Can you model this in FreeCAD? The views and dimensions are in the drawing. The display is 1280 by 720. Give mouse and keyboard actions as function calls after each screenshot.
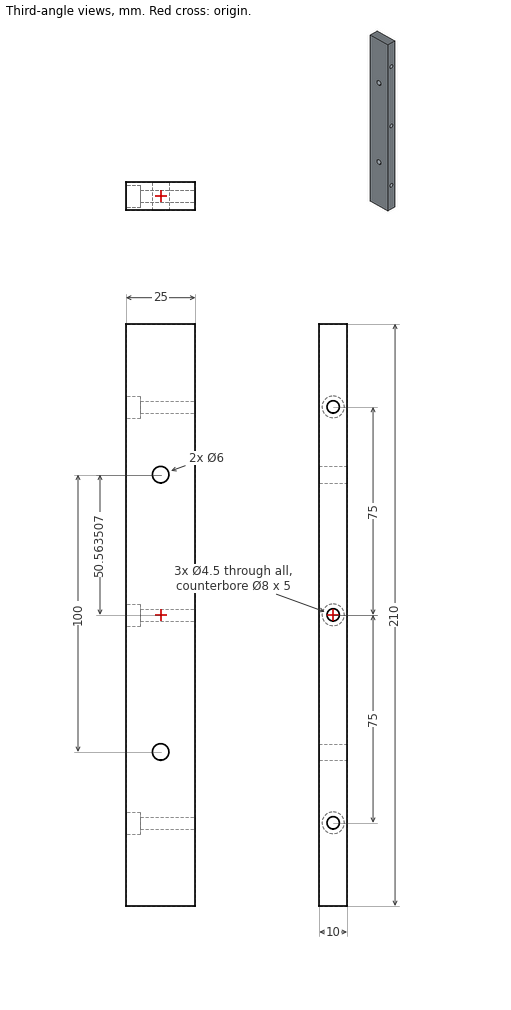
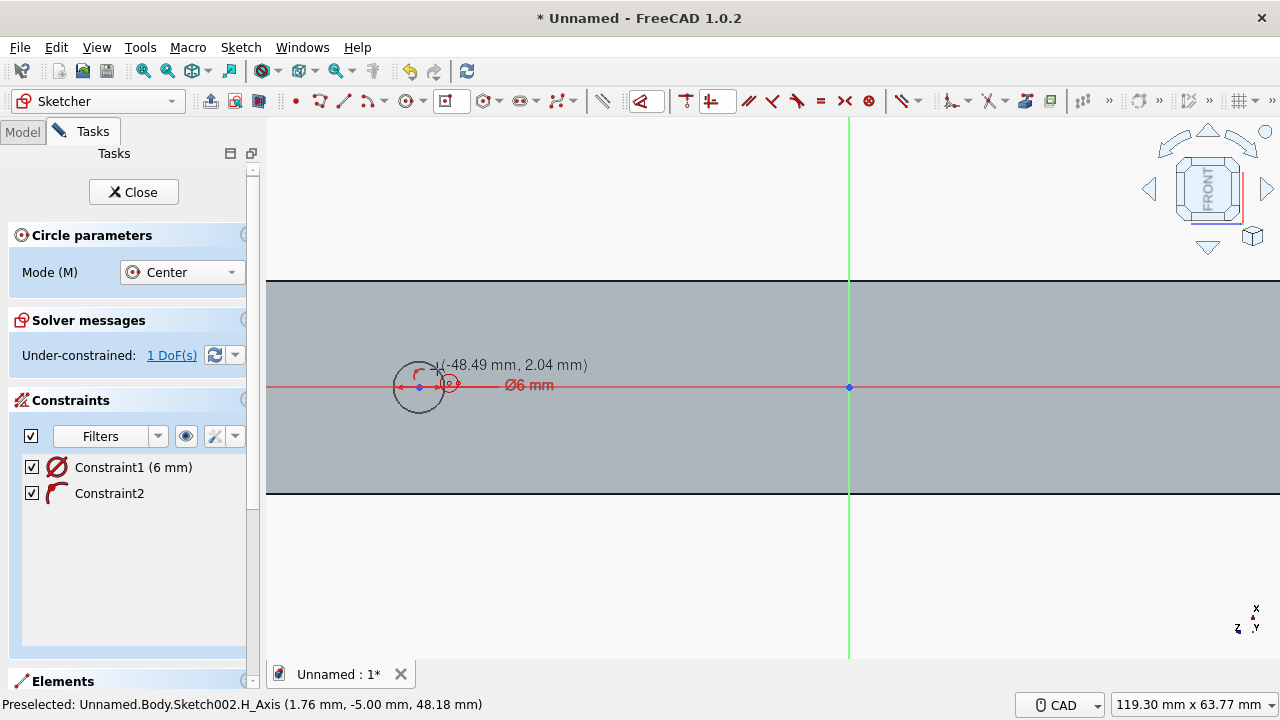
scroll(420, 389, down, 2)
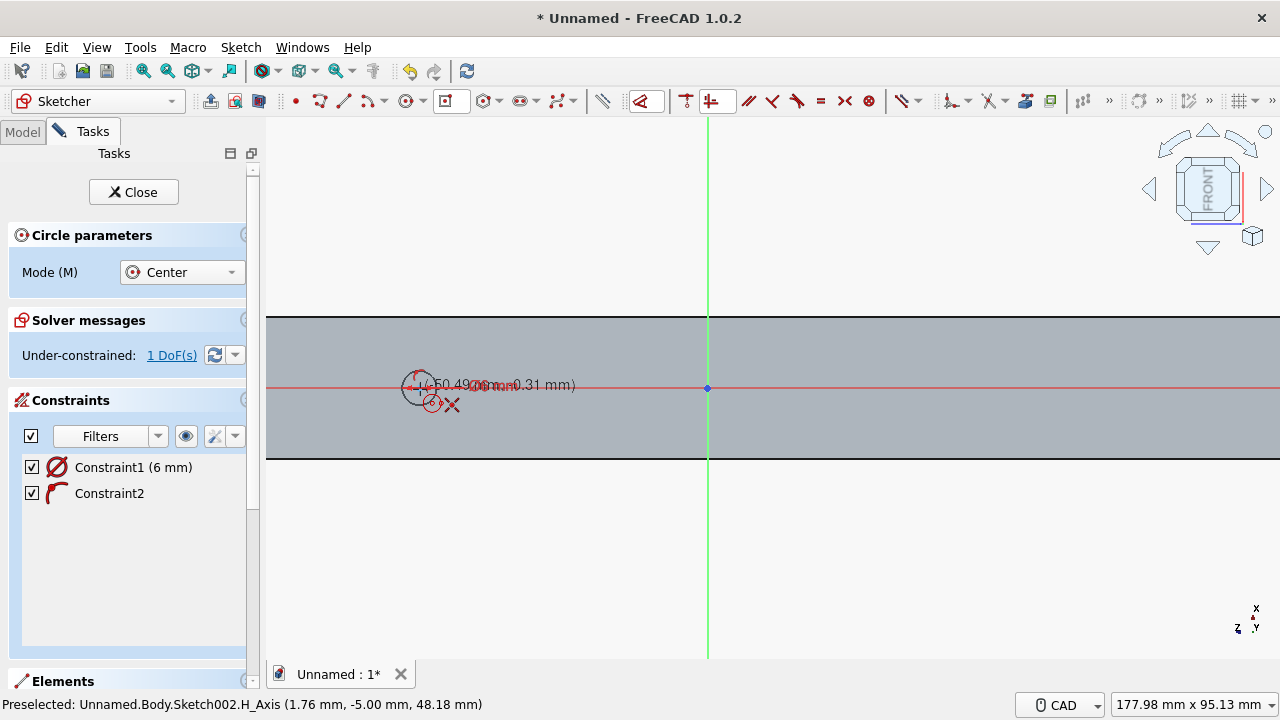
scroll(989, 388, up, 2)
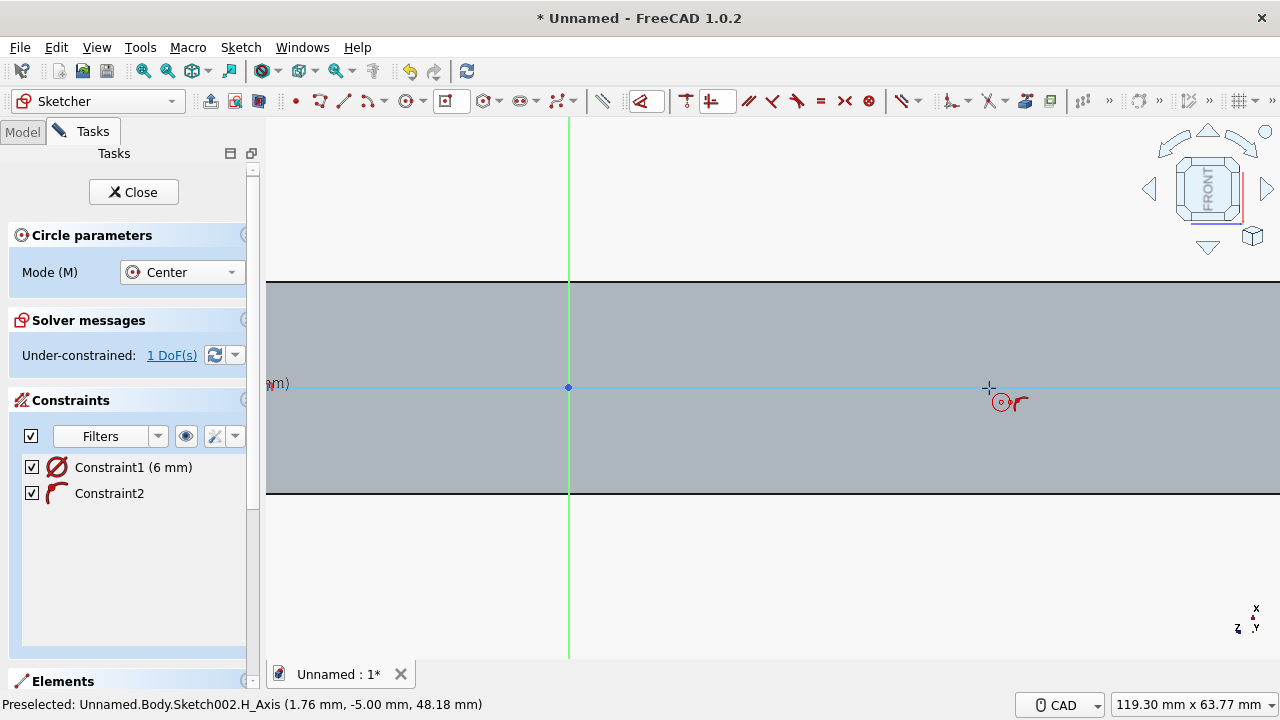
click(989, 388)
move(1007, 370)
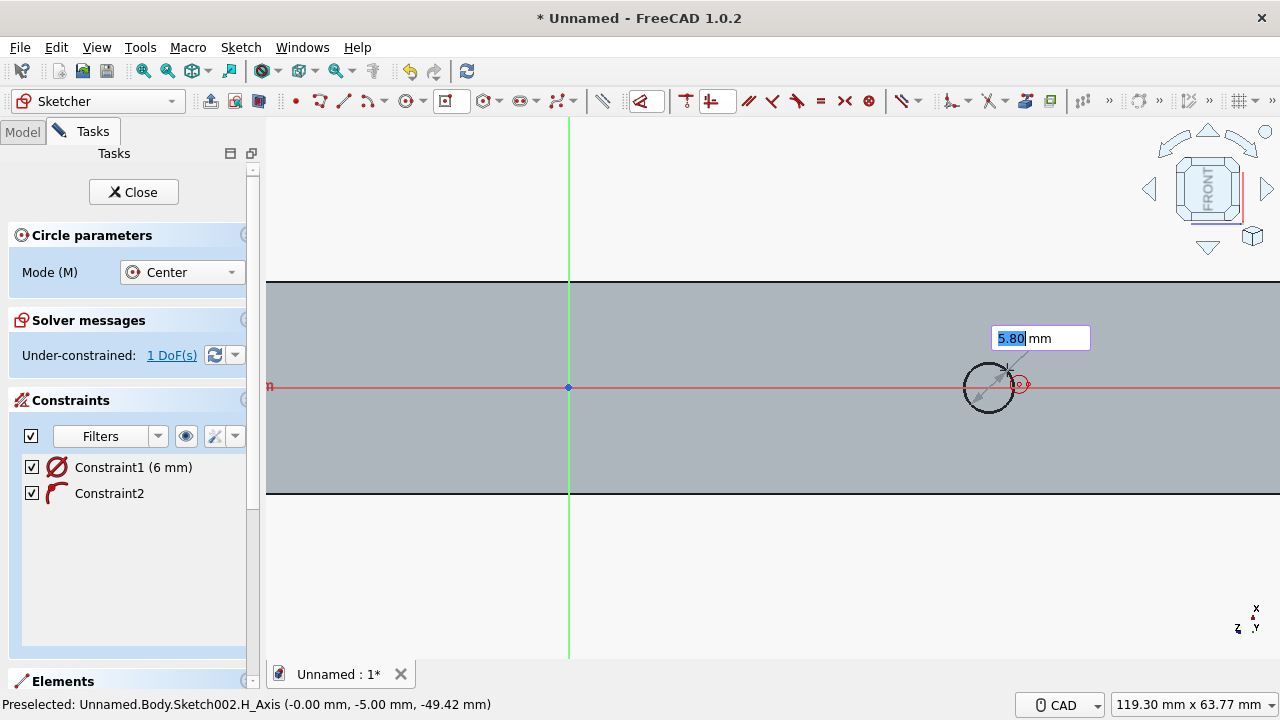
text(6)
key(Return)
key(Escape)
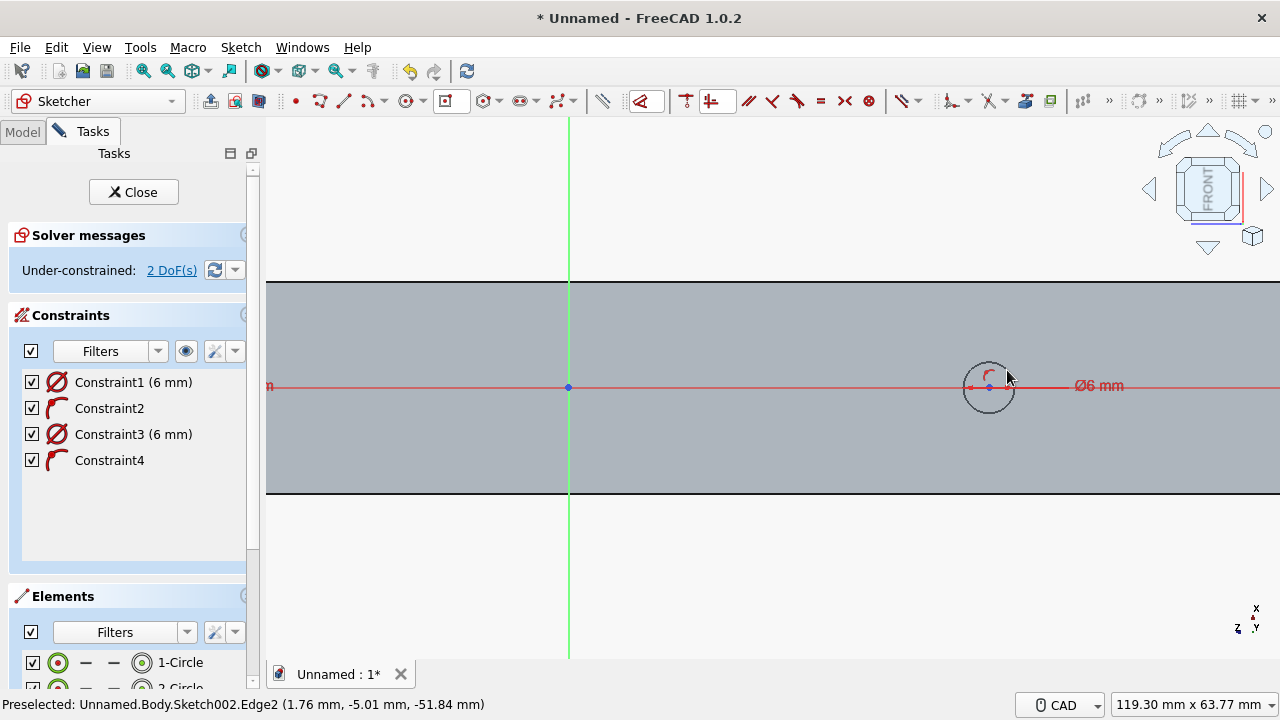
scroll(990, 388, down, 2)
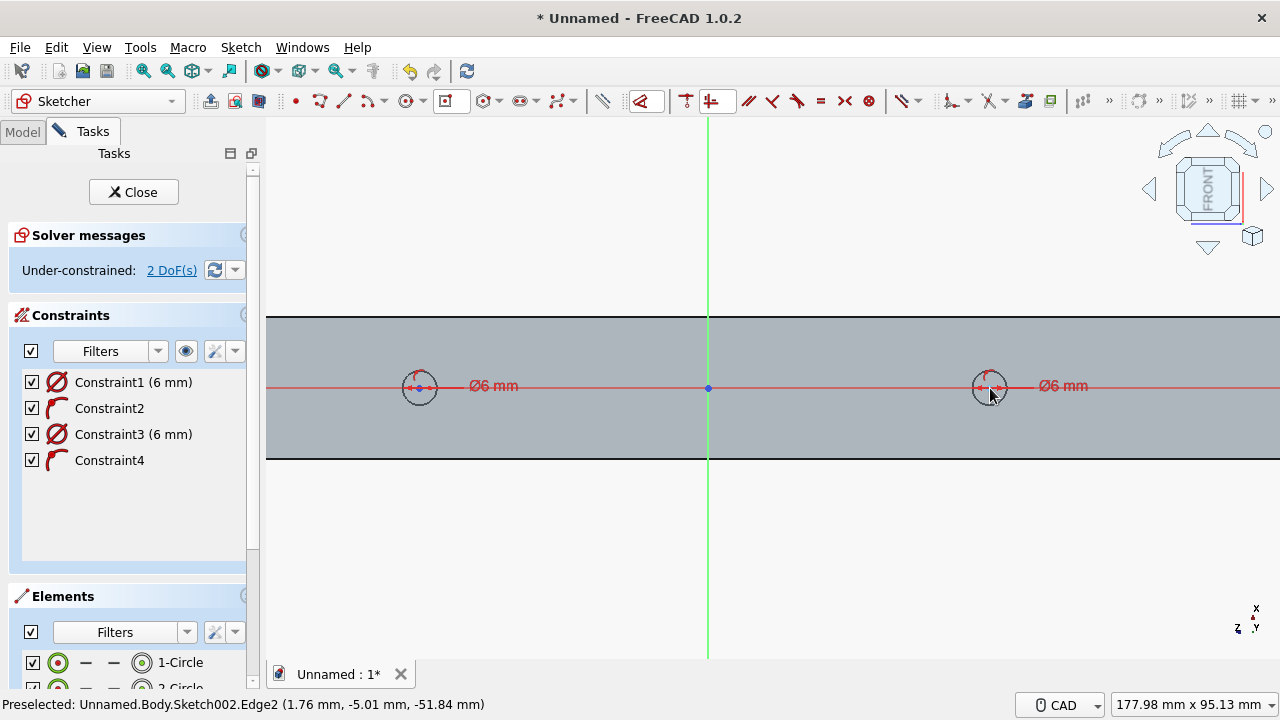
click(420, 388)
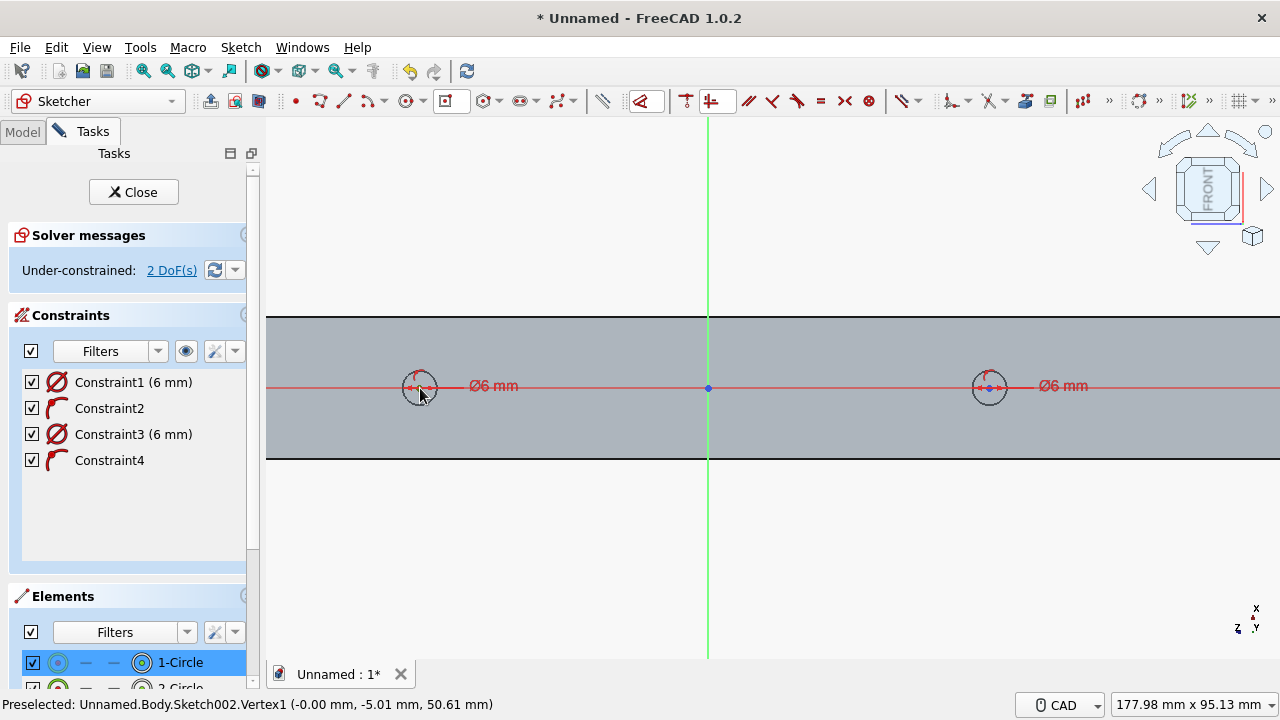
click(990, 388)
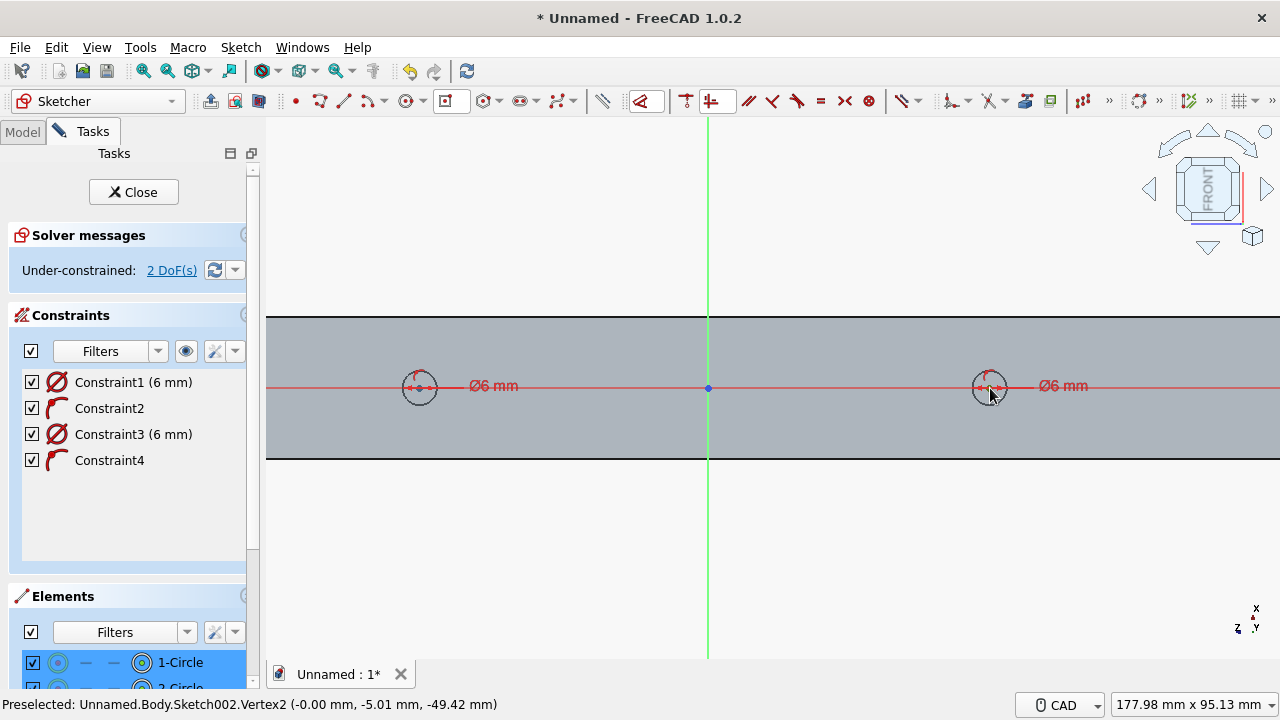
key(l)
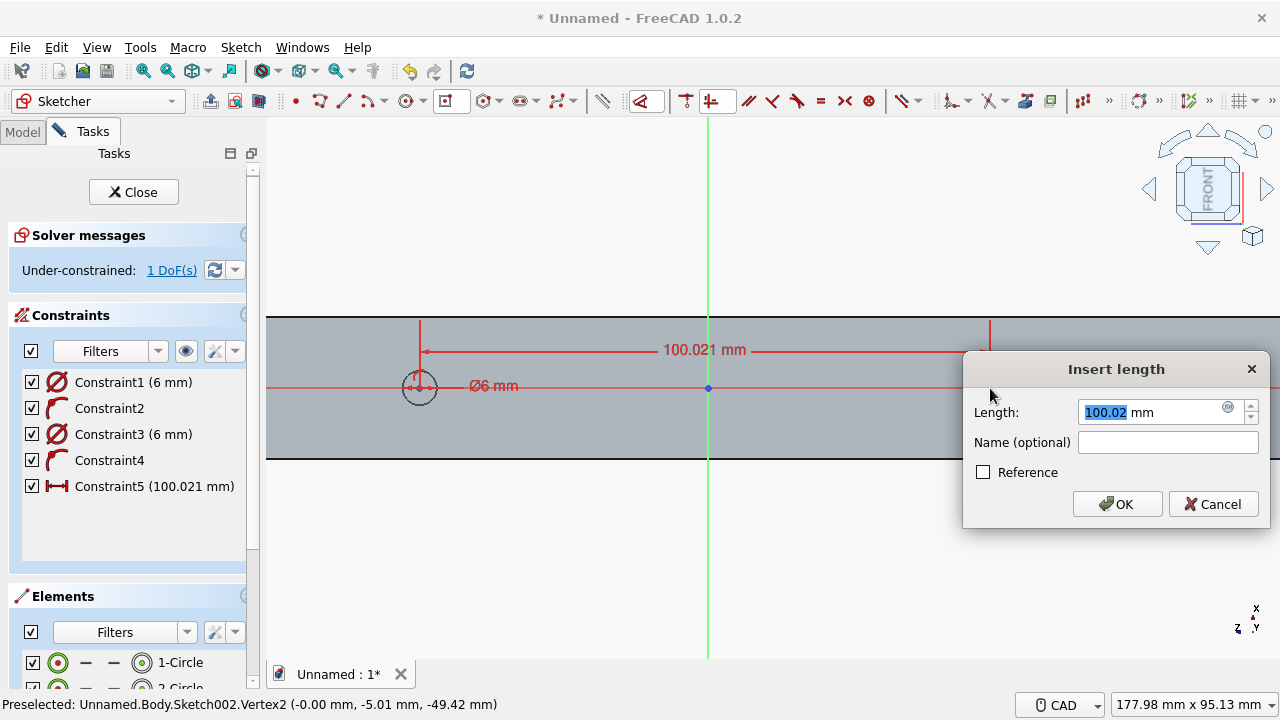
text(100)
key(Return)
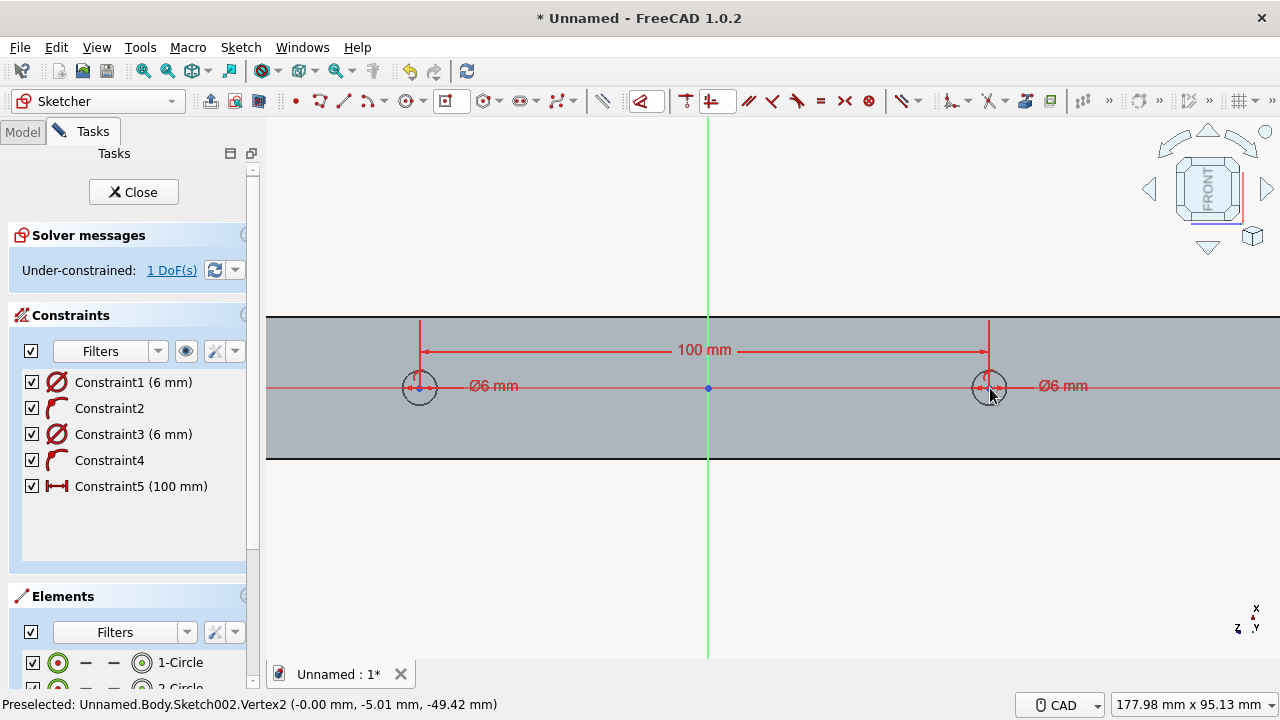
click(420, 388)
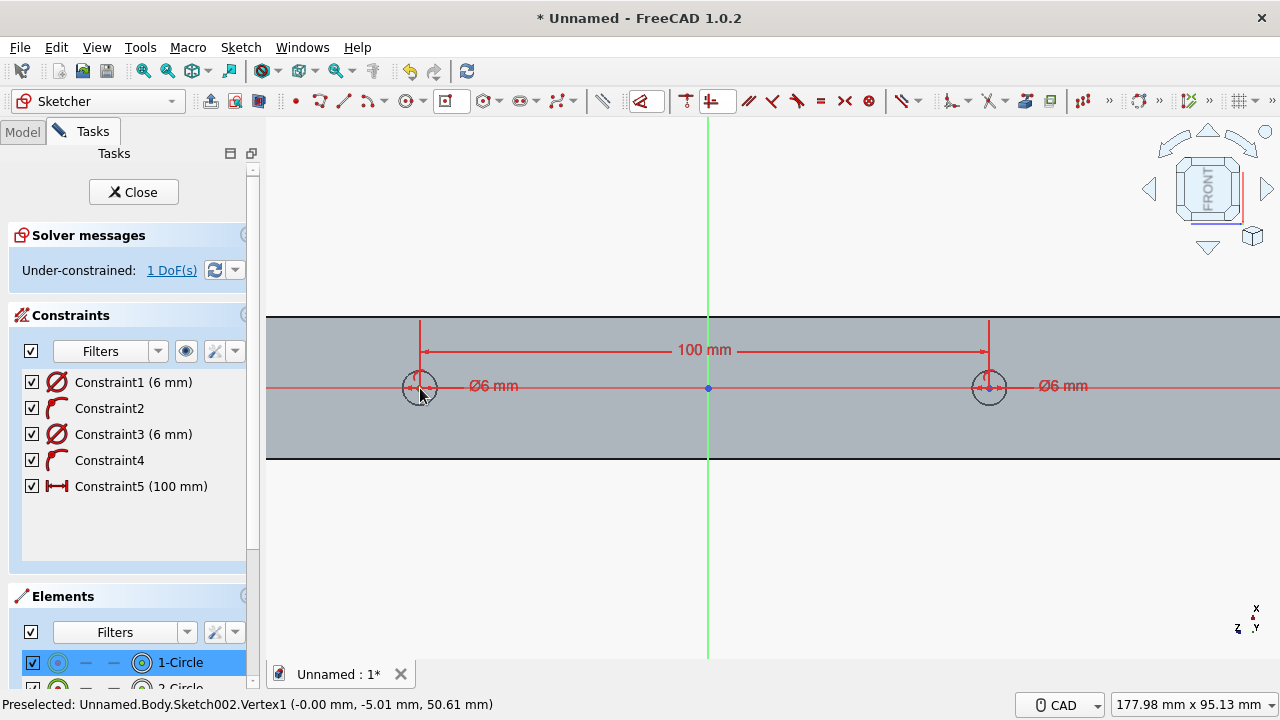
key(l)